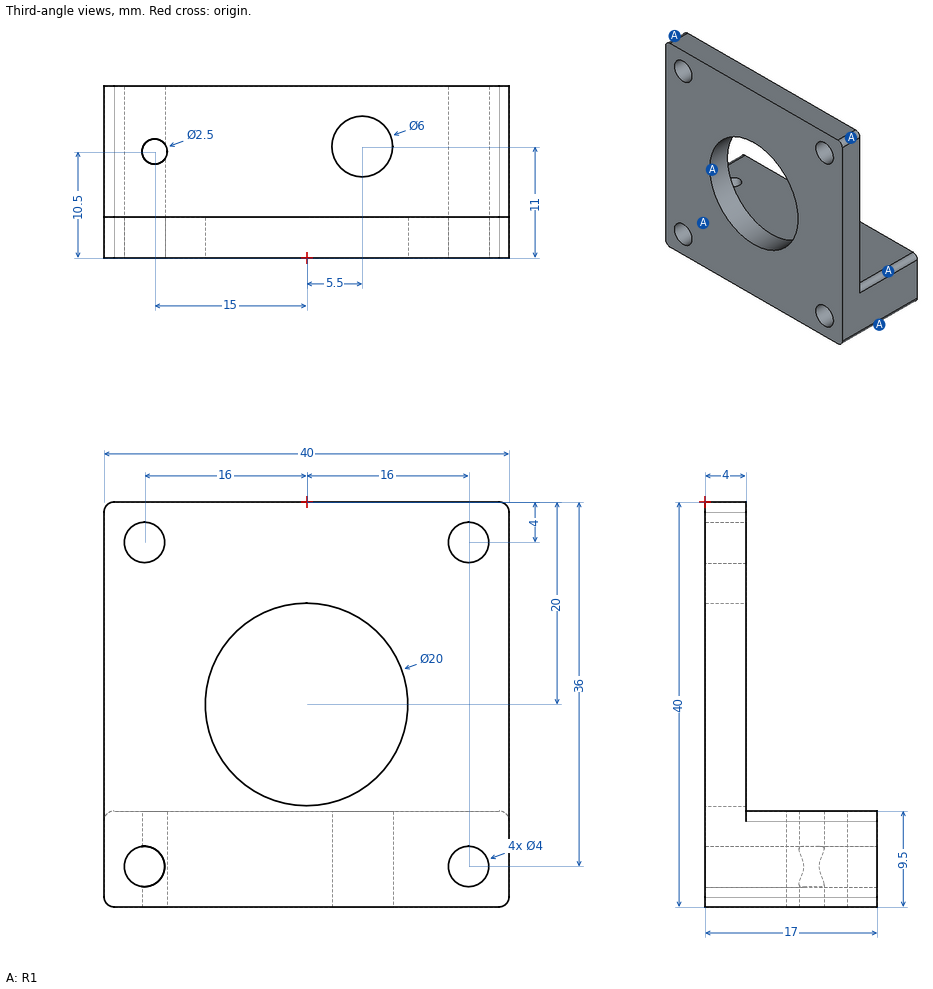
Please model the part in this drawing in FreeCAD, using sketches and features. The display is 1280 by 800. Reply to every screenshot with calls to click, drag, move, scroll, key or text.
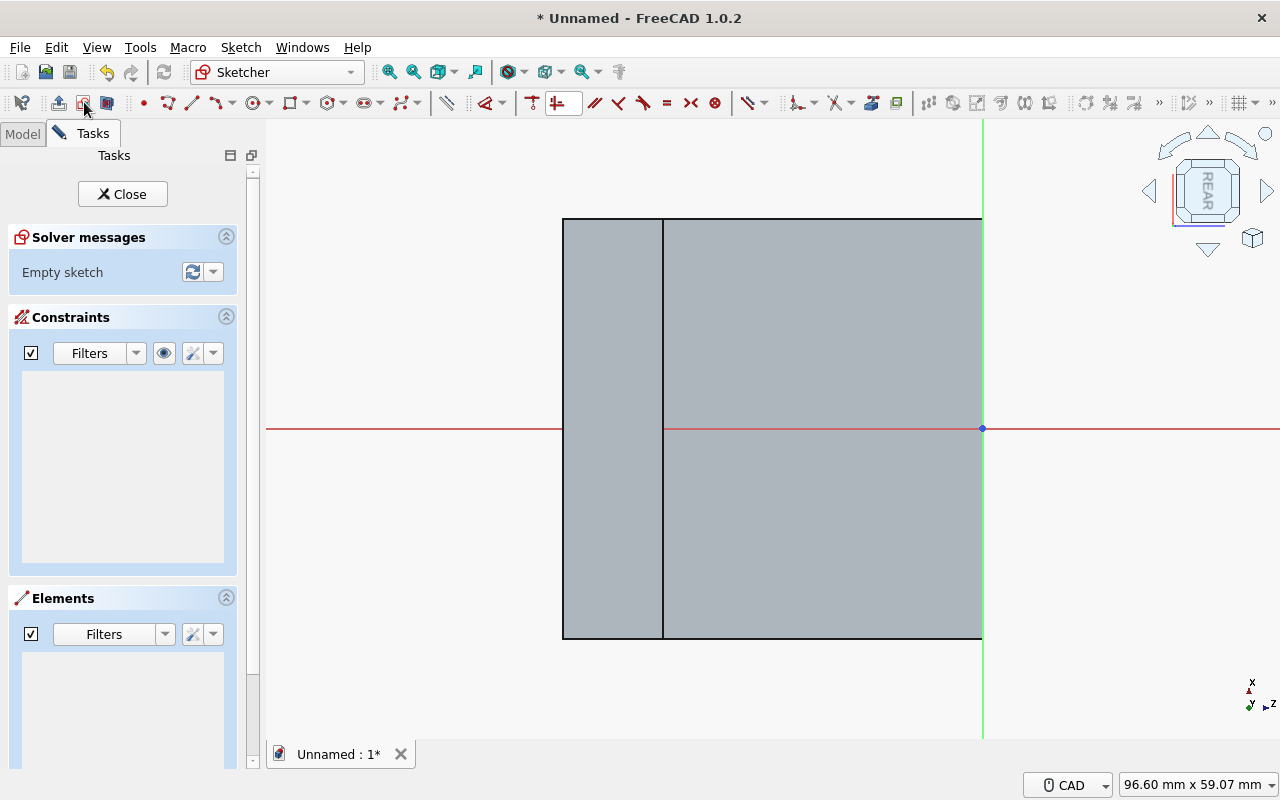
key(g)
key(c)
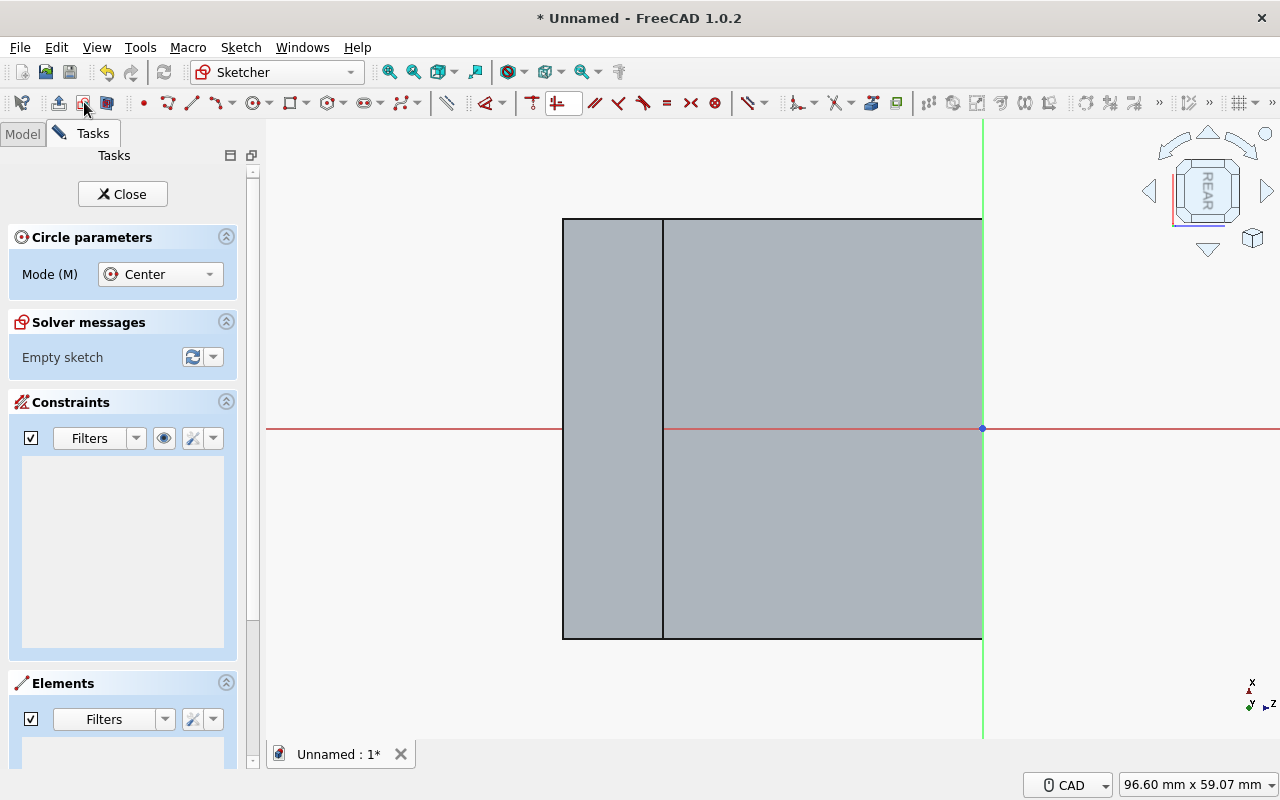
click(773, 429)
move(847, 355)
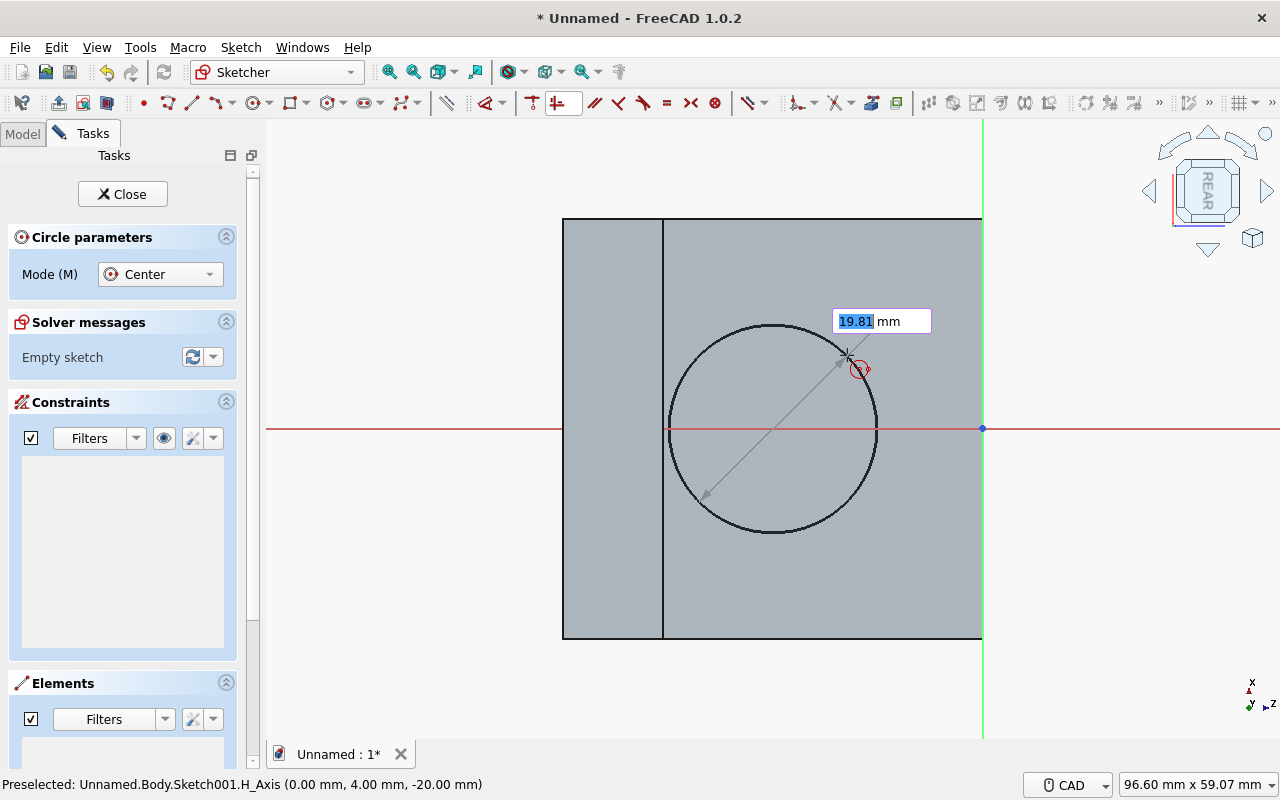
text(20)
key(Return)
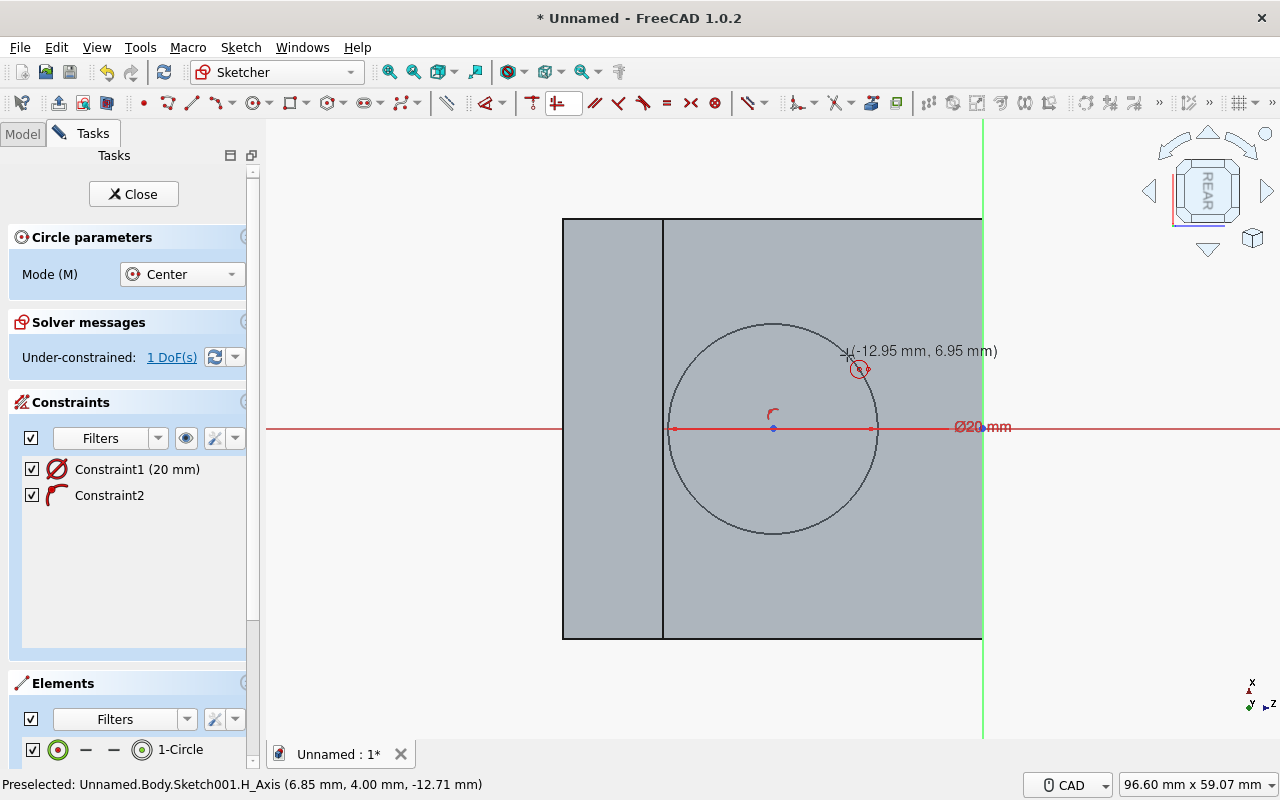
click(605, 261)
move(620, 246)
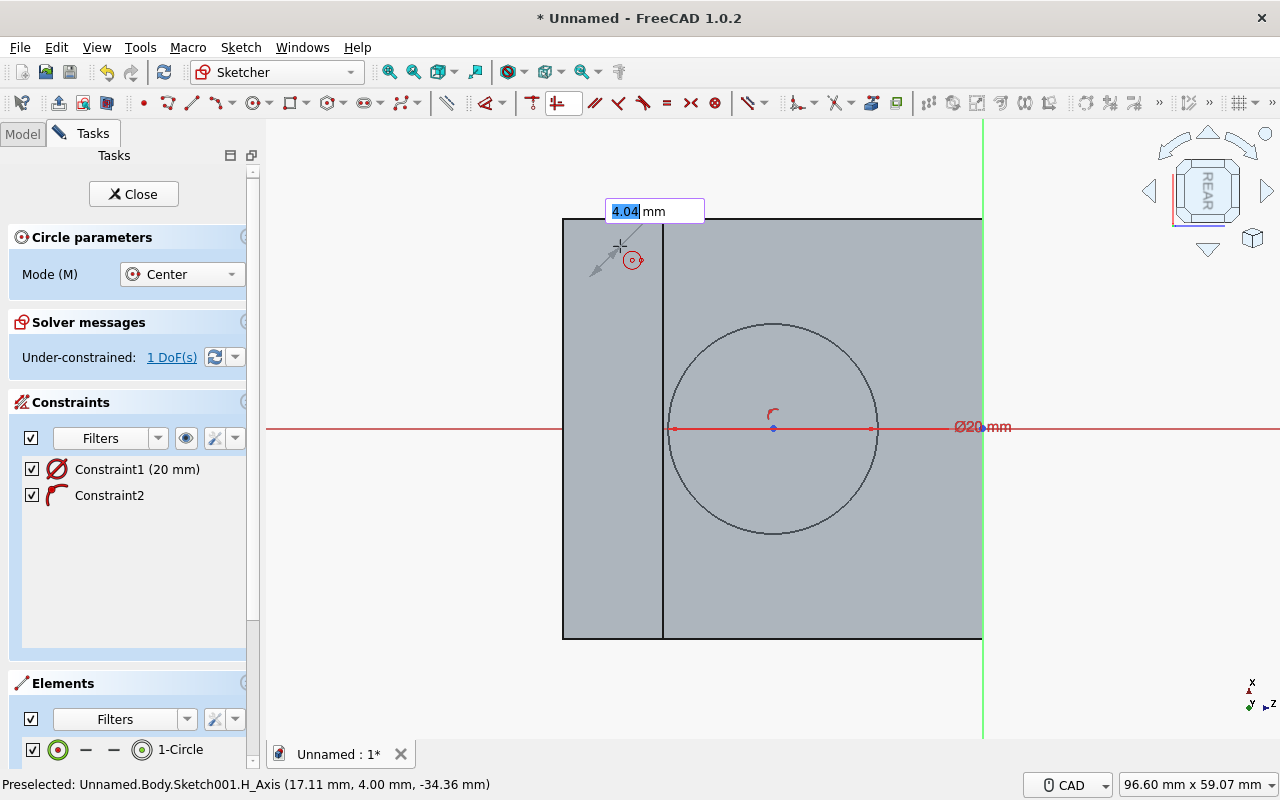
text(4)
key(Return)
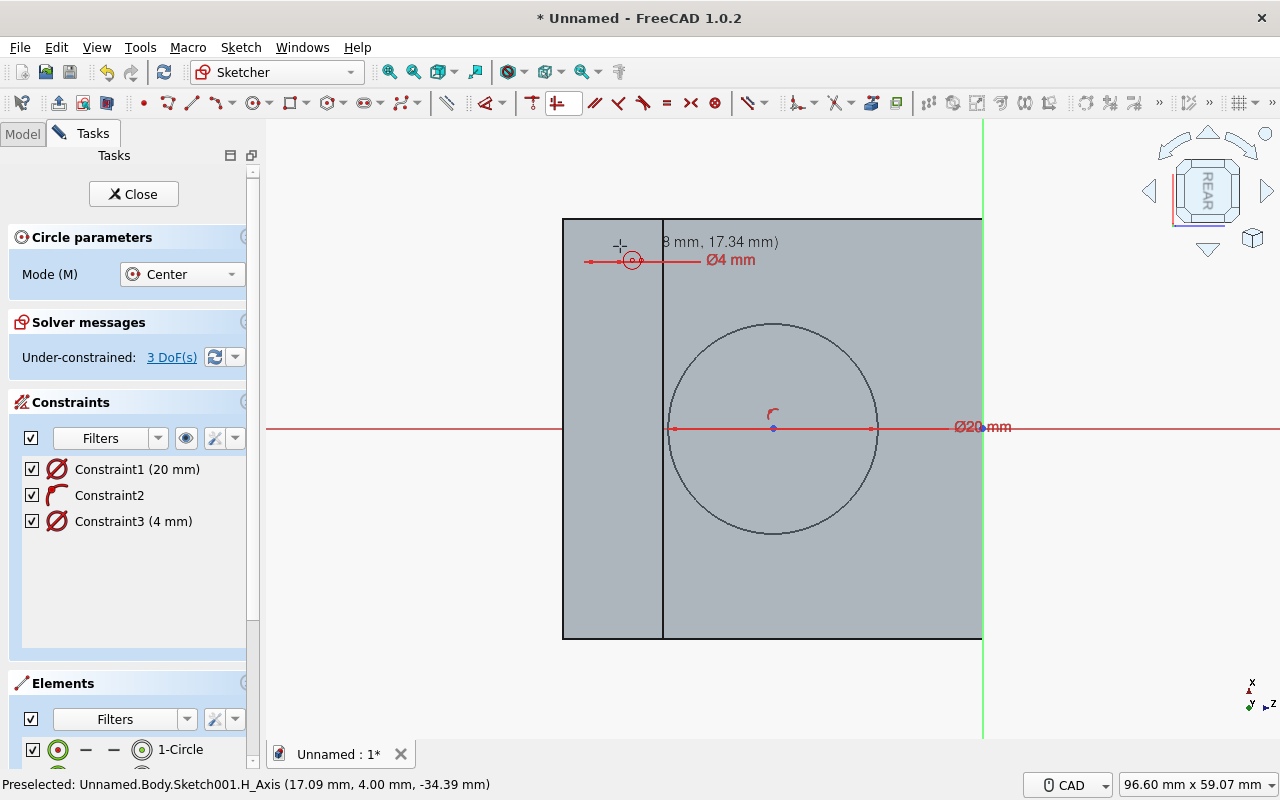
click(941, 261)
move(956, 246)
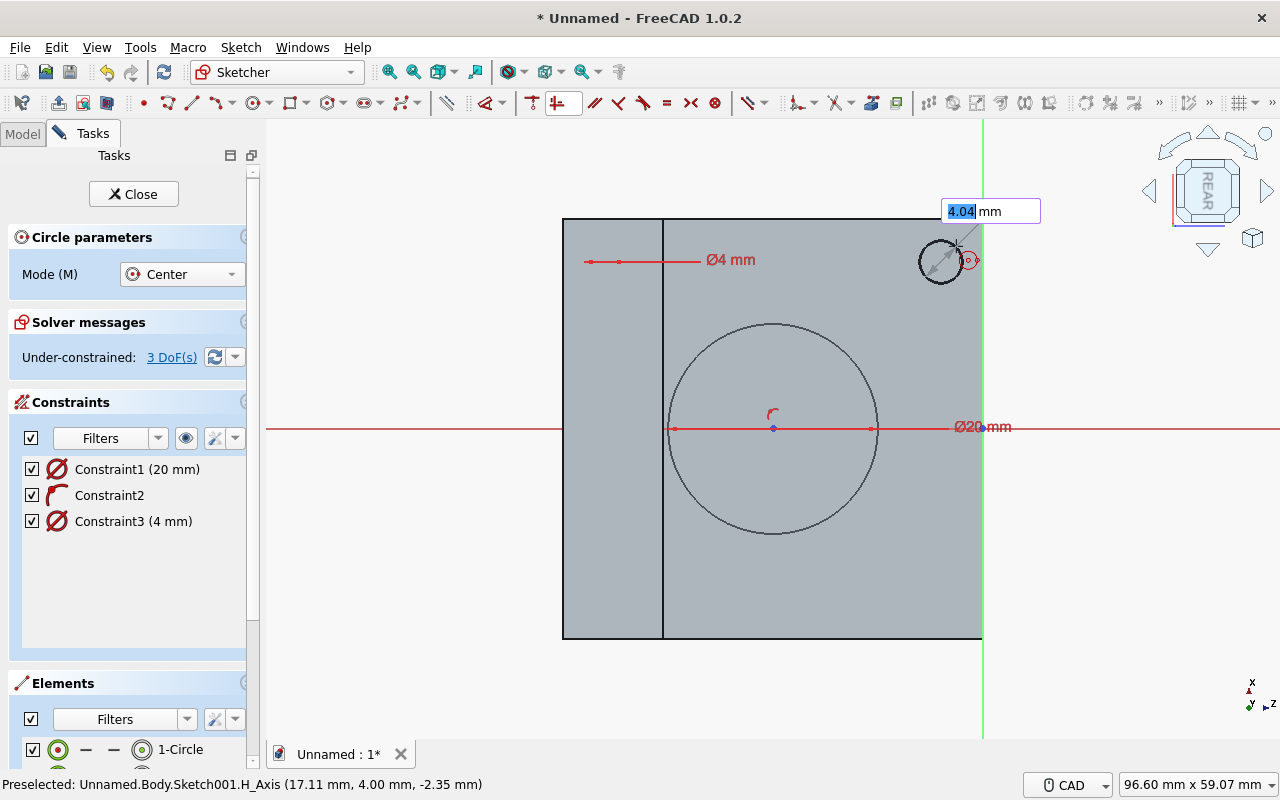
text(4)
key(Return)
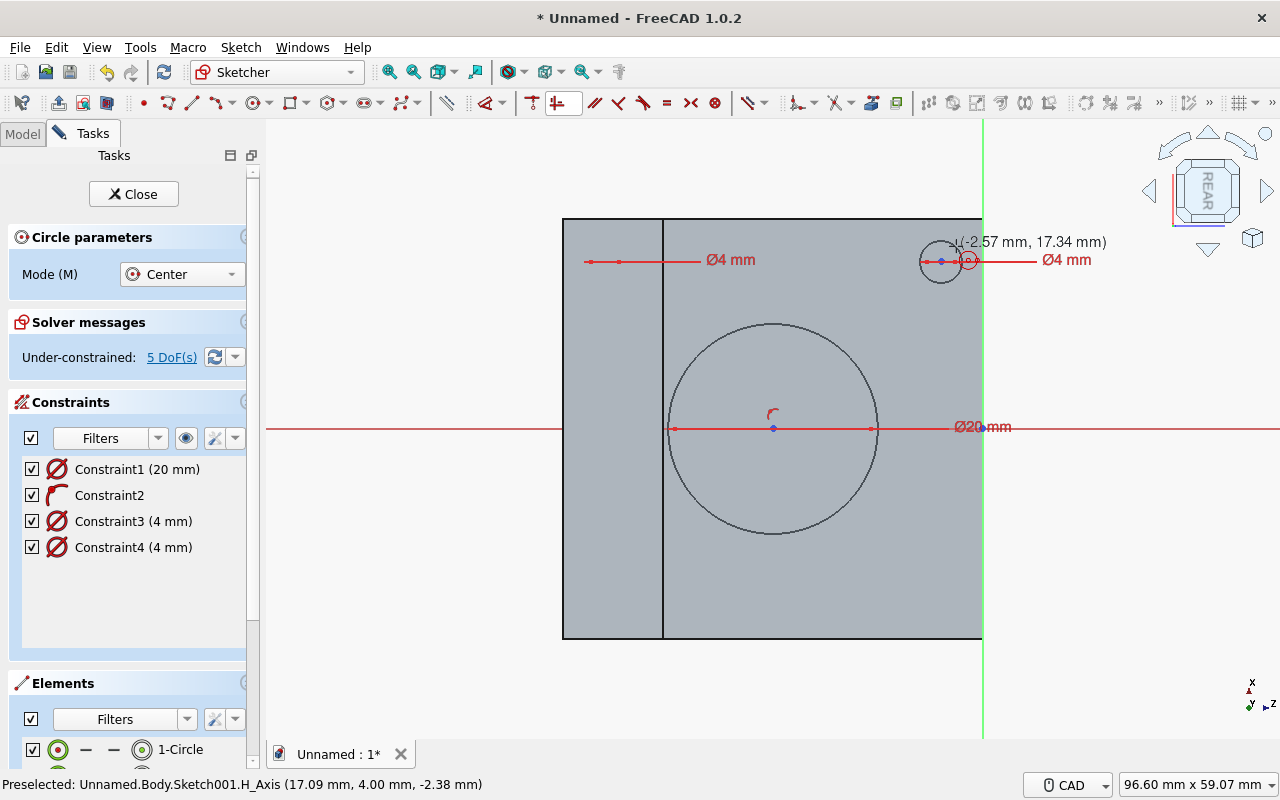
click(941, 597)
move(956, 582)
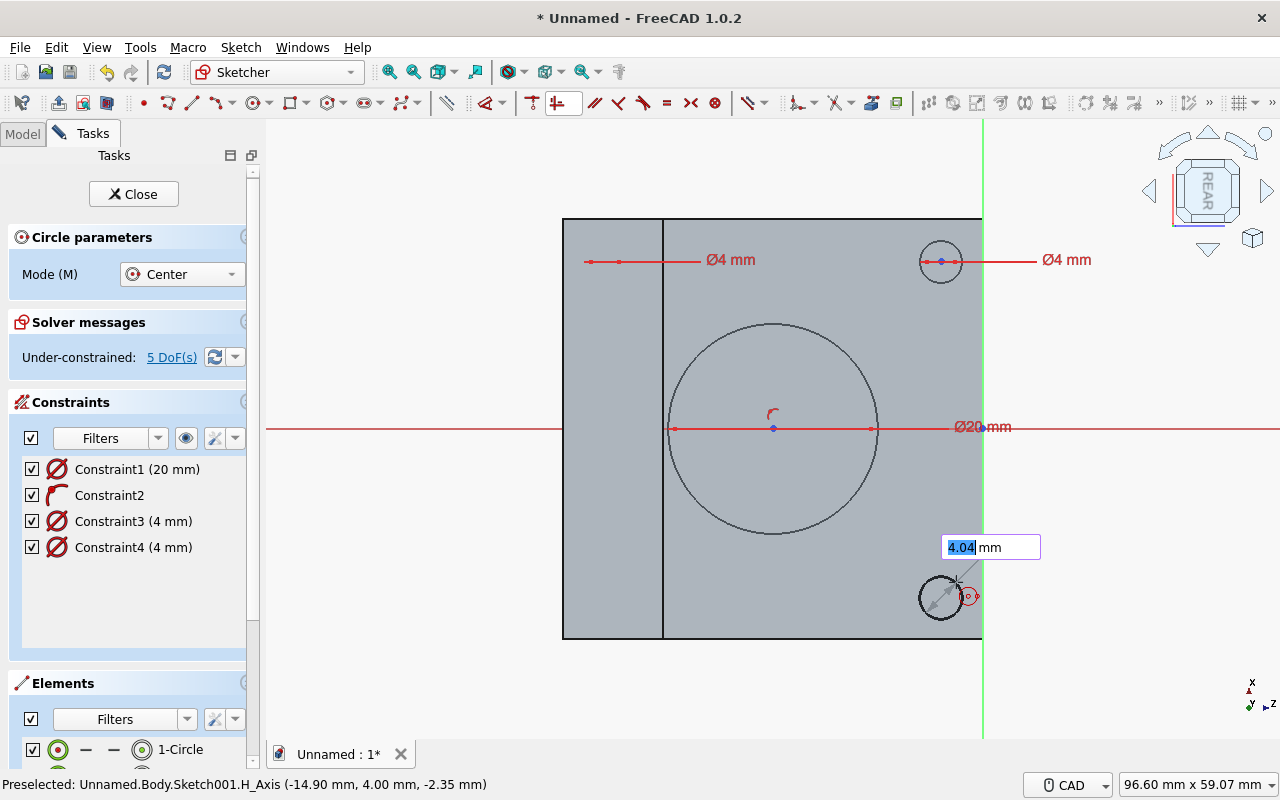
text(4)
key(Return)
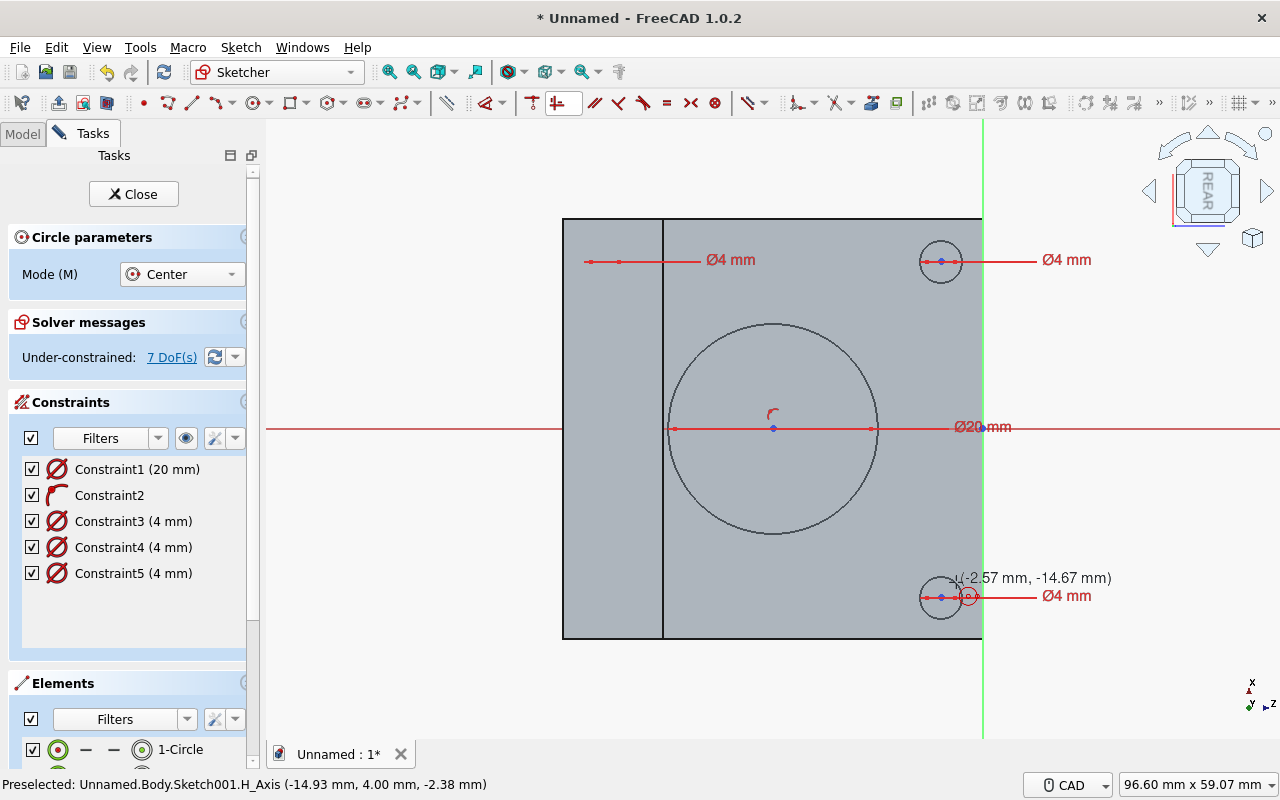
click(605, 597)
move(620, 582)